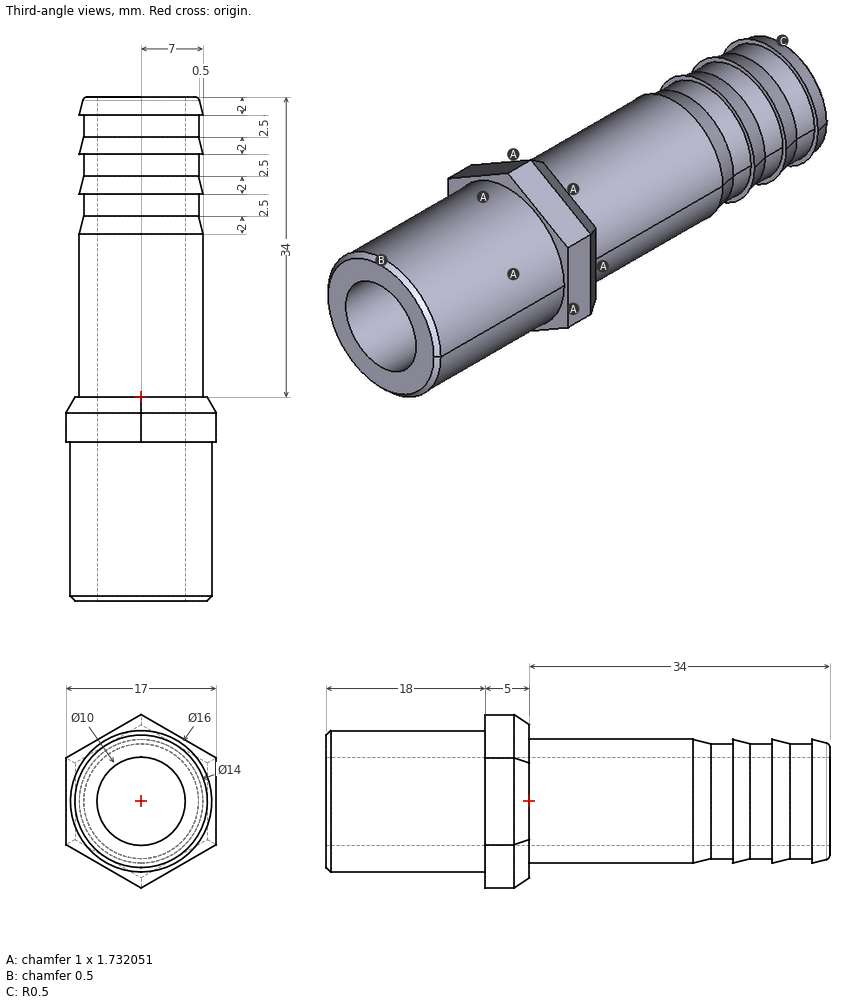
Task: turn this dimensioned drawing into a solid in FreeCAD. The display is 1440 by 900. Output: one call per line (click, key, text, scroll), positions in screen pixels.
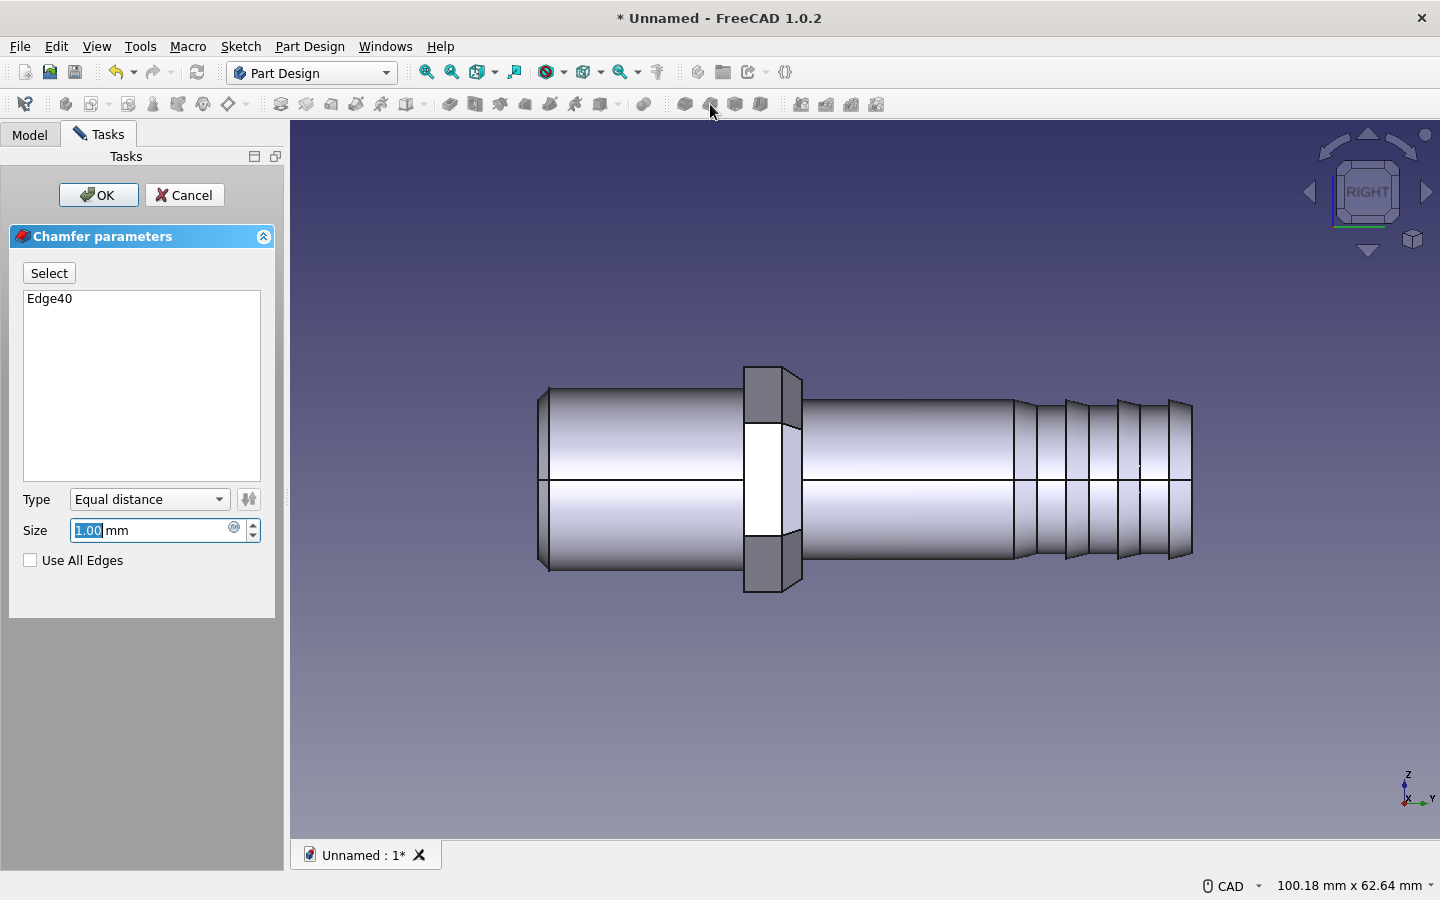
text(0.5)
key(Tab)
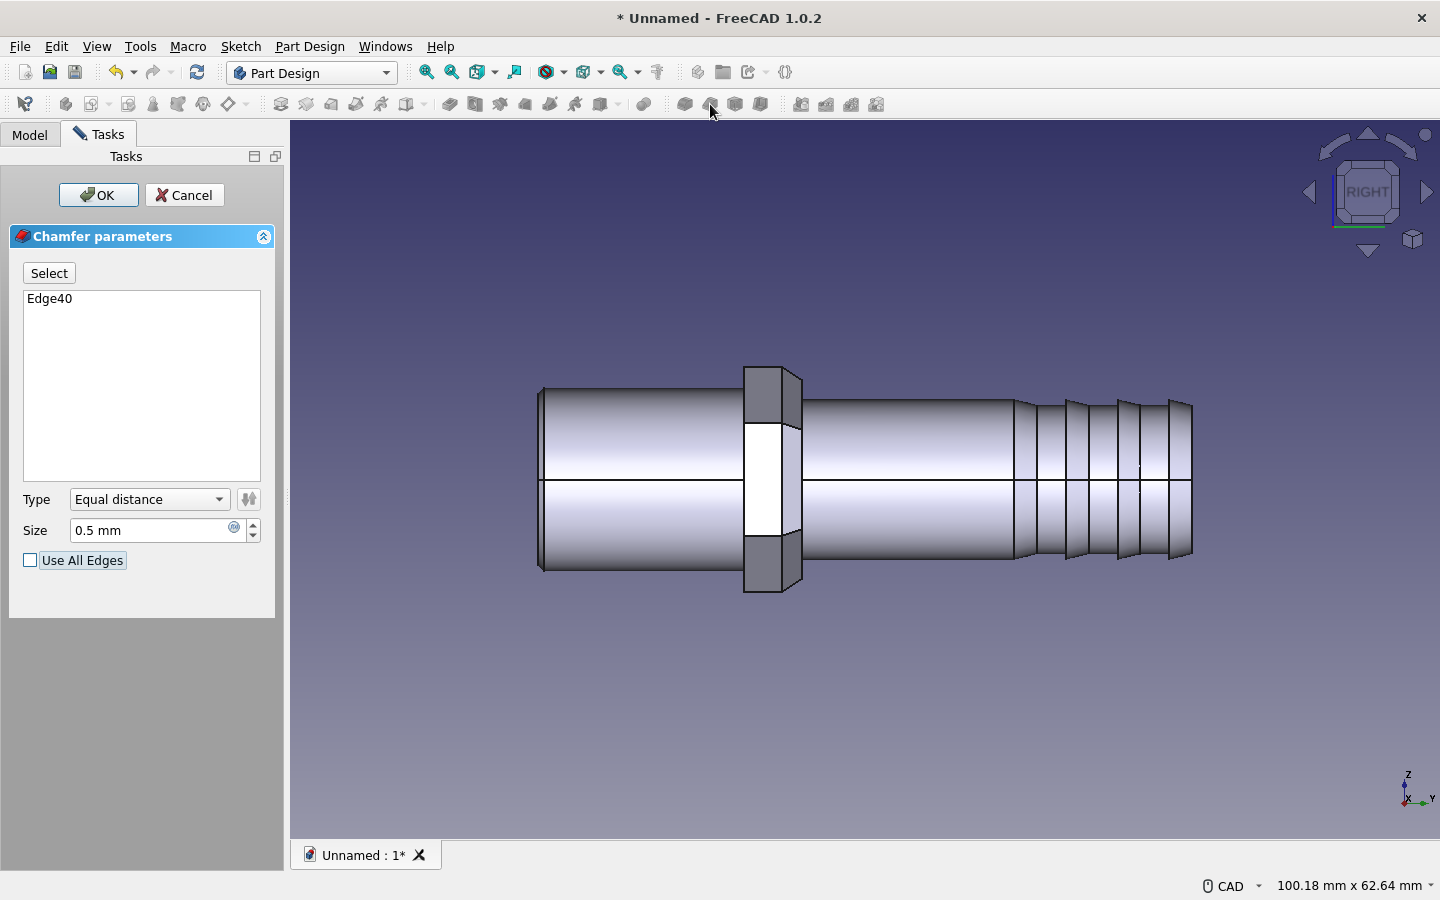
click(99, 195)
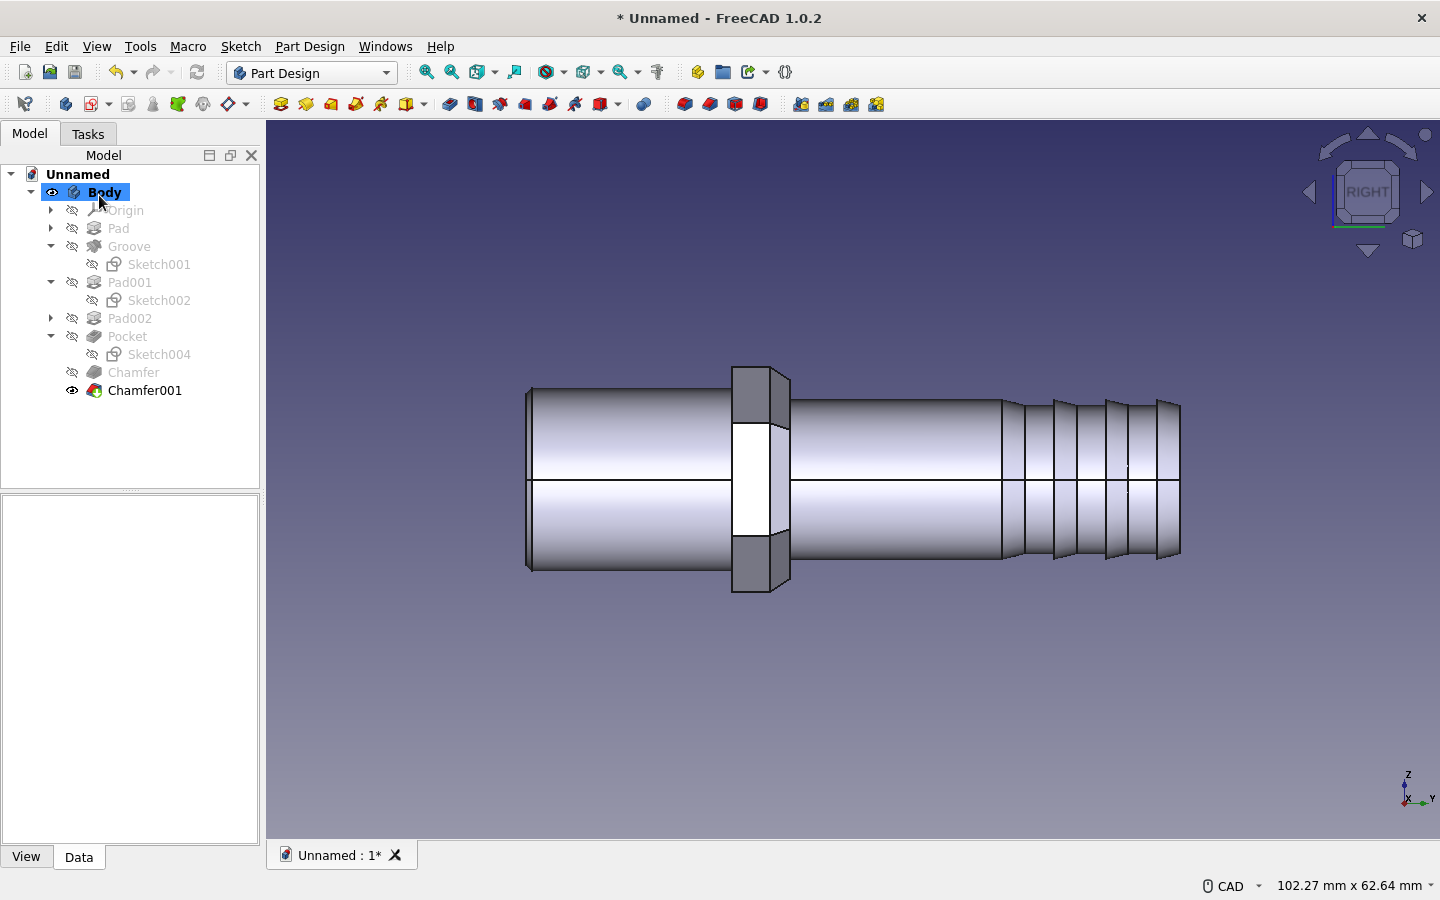
click(1180, 522)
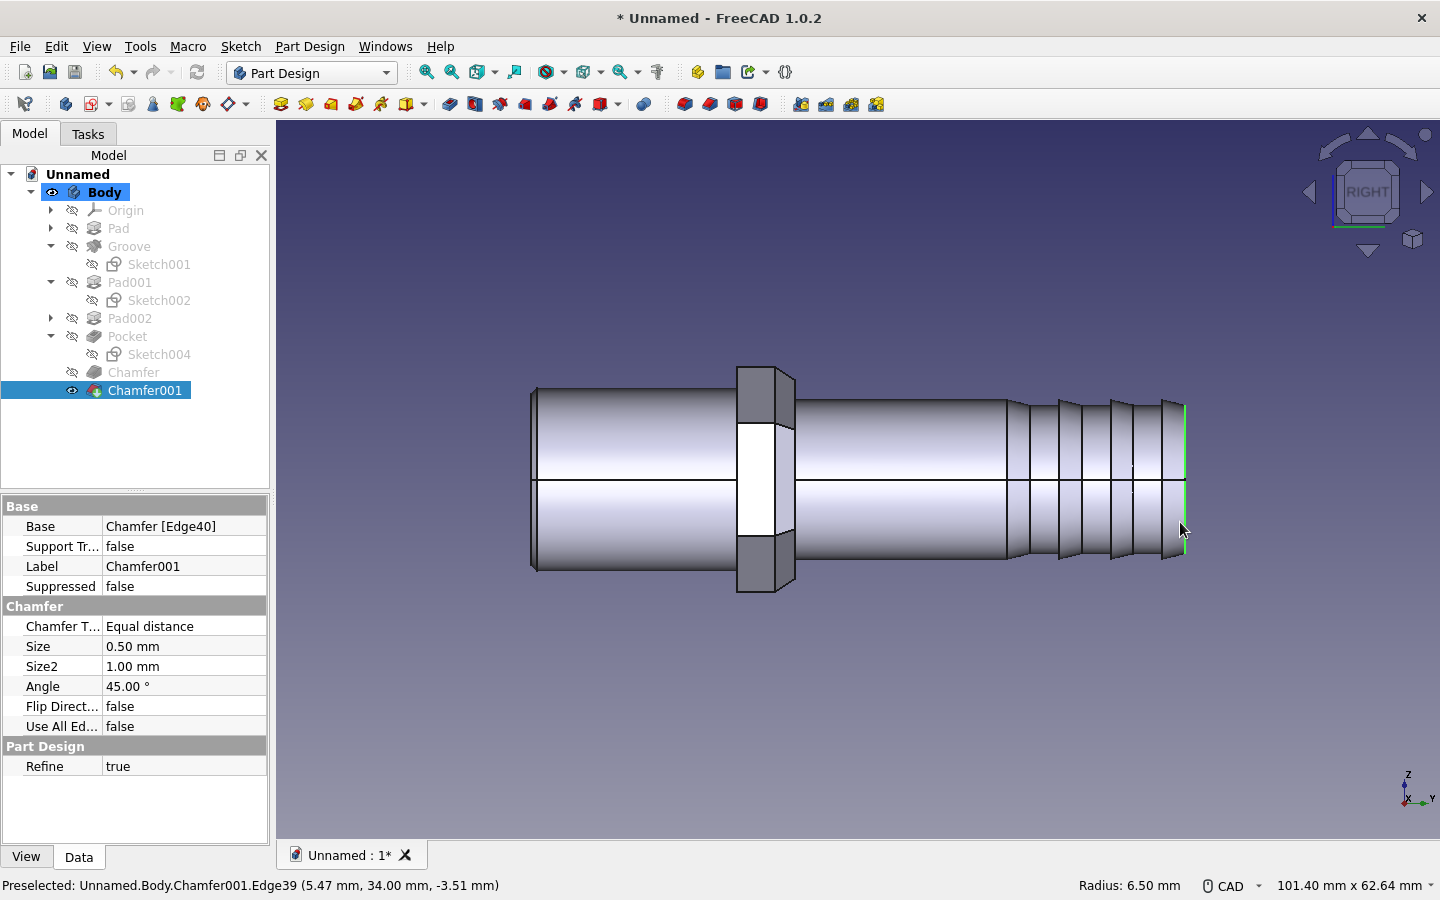
click(685, 104)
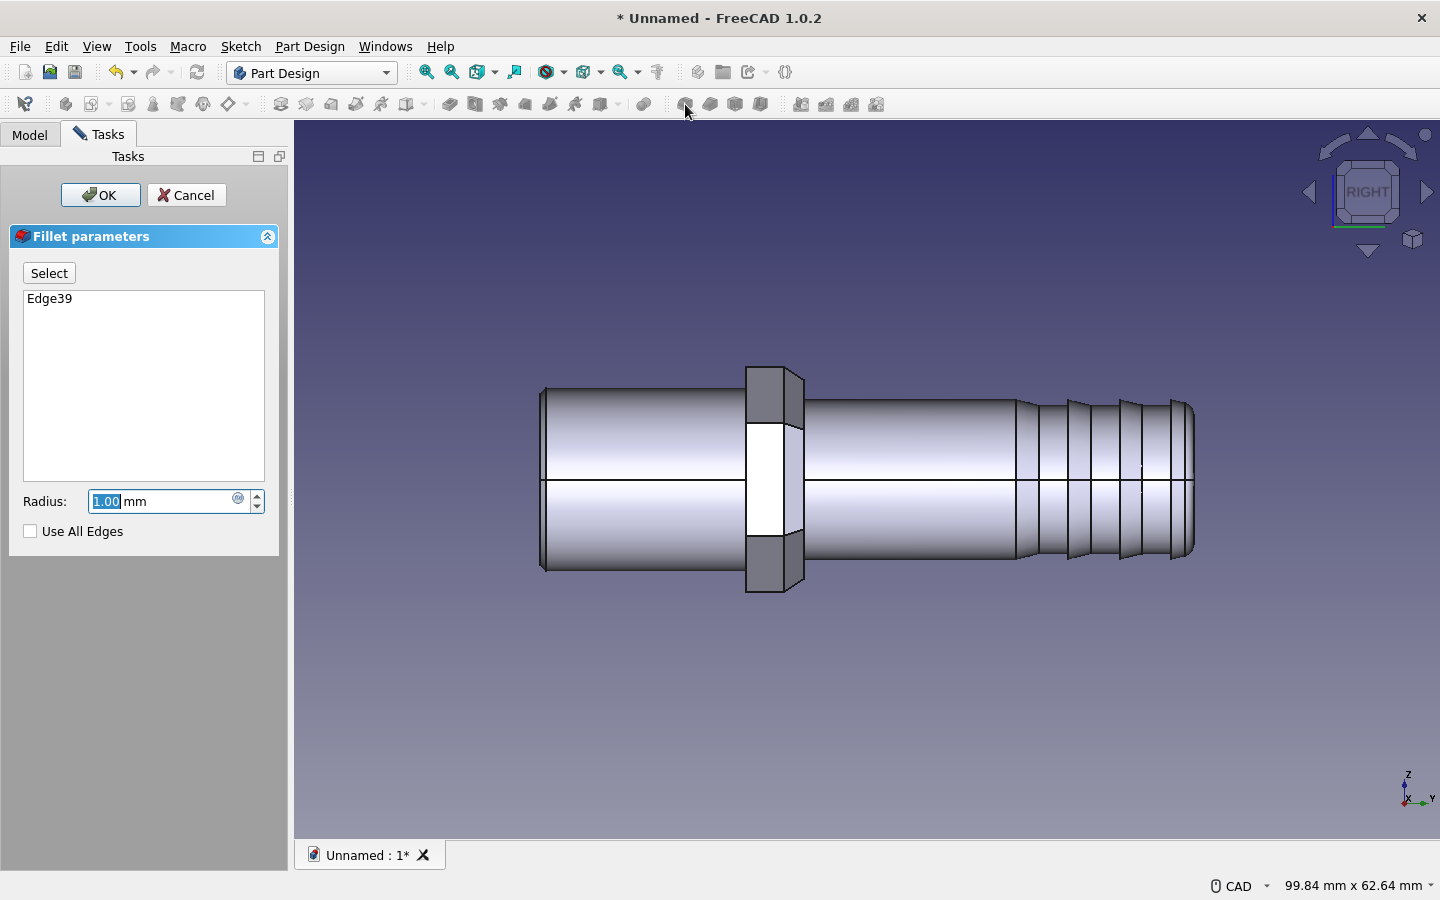
text(0.5)
key(Tab)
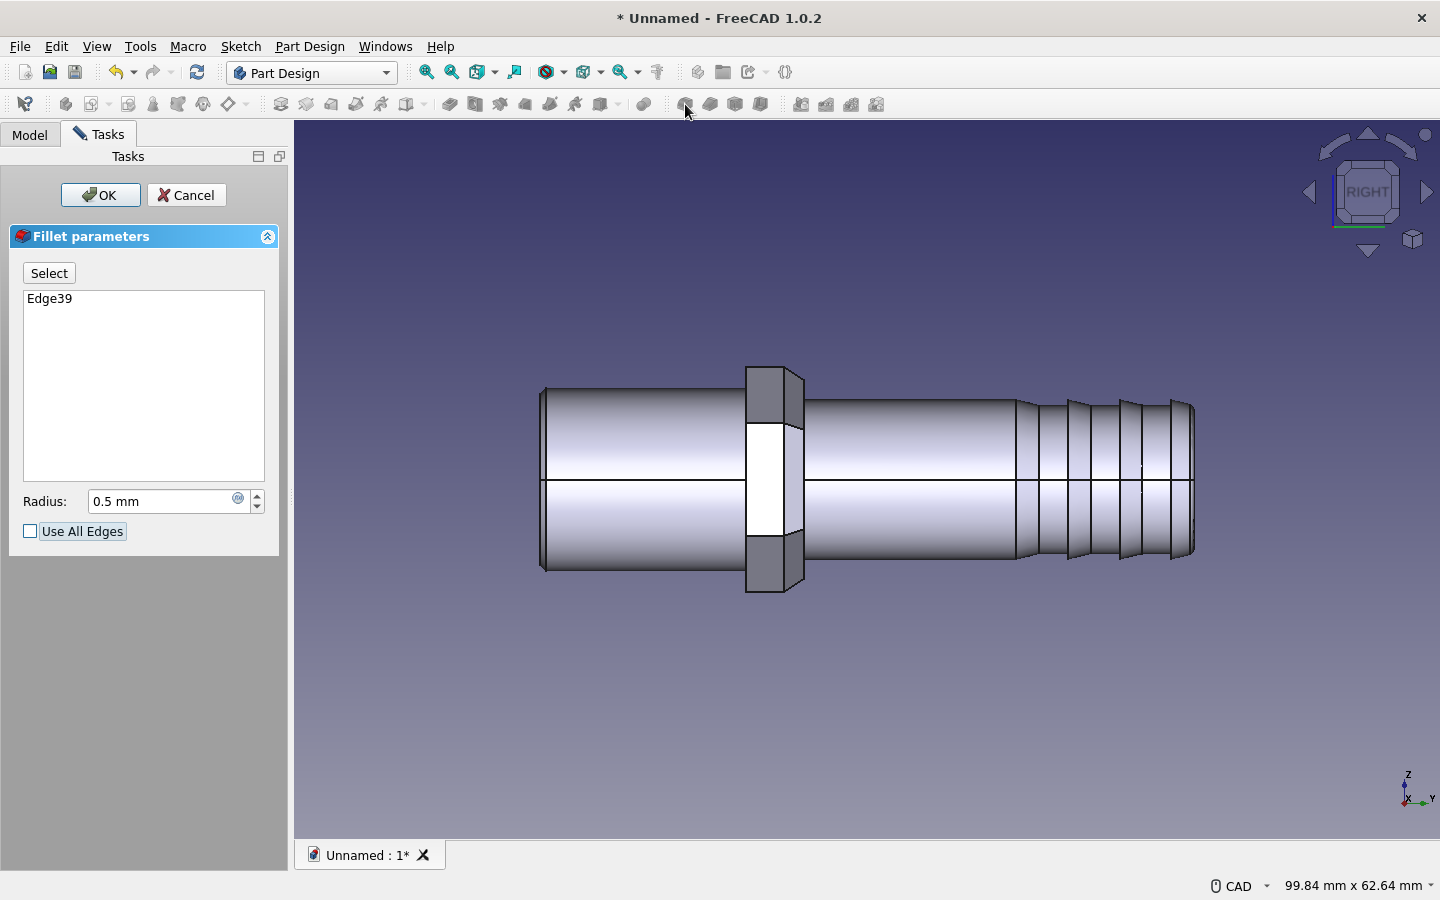
click(101, 195)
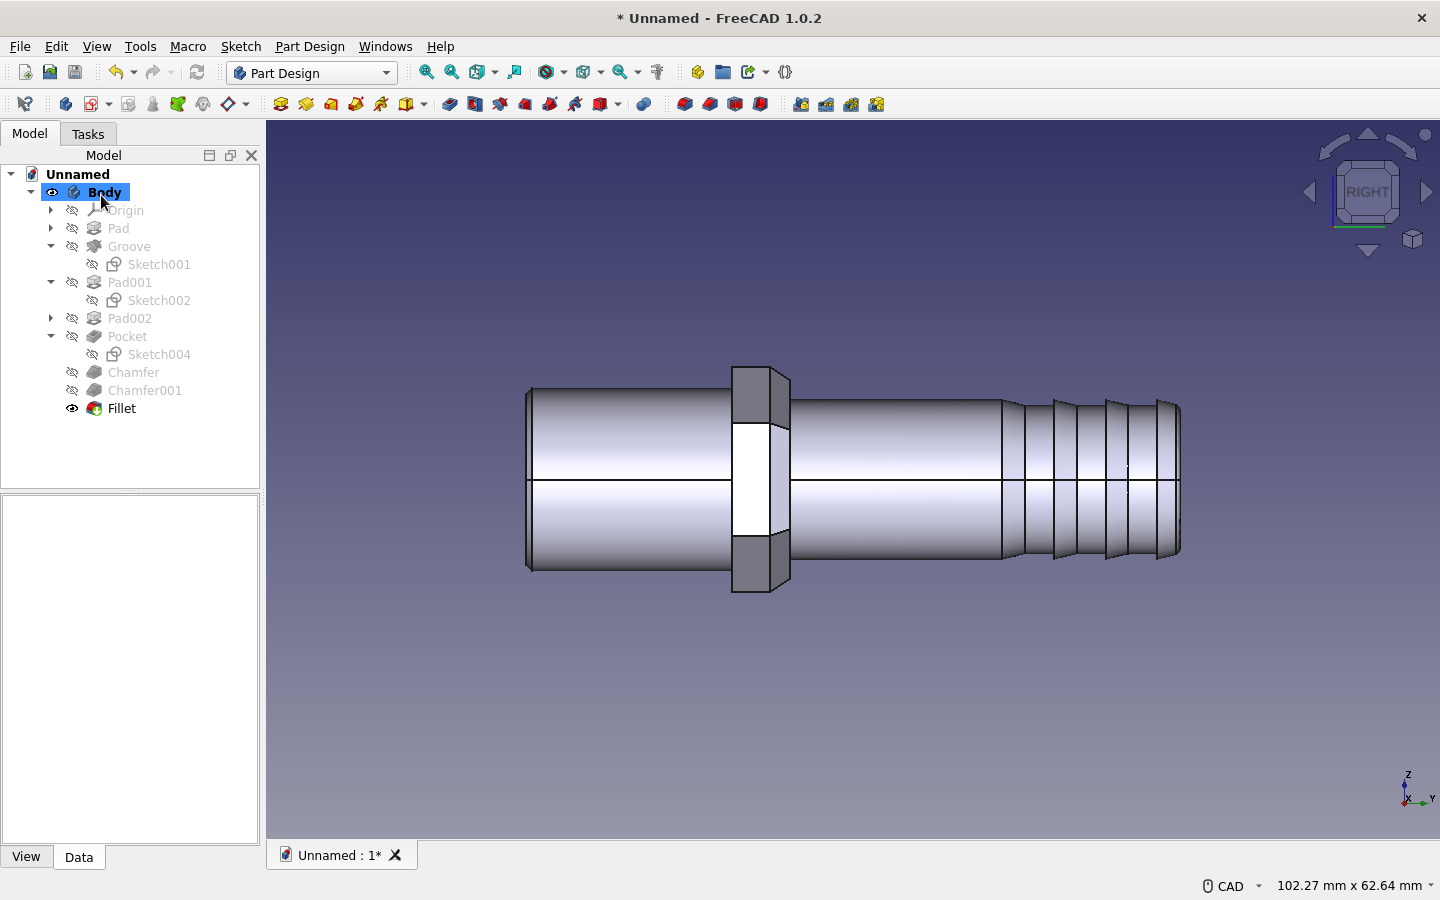
key(0)